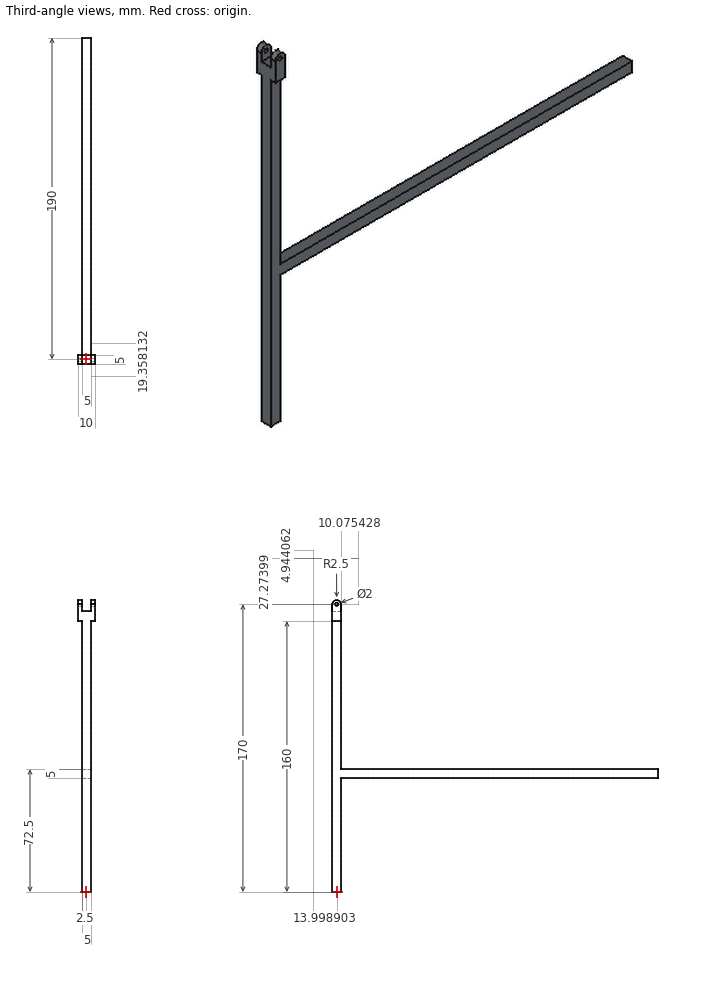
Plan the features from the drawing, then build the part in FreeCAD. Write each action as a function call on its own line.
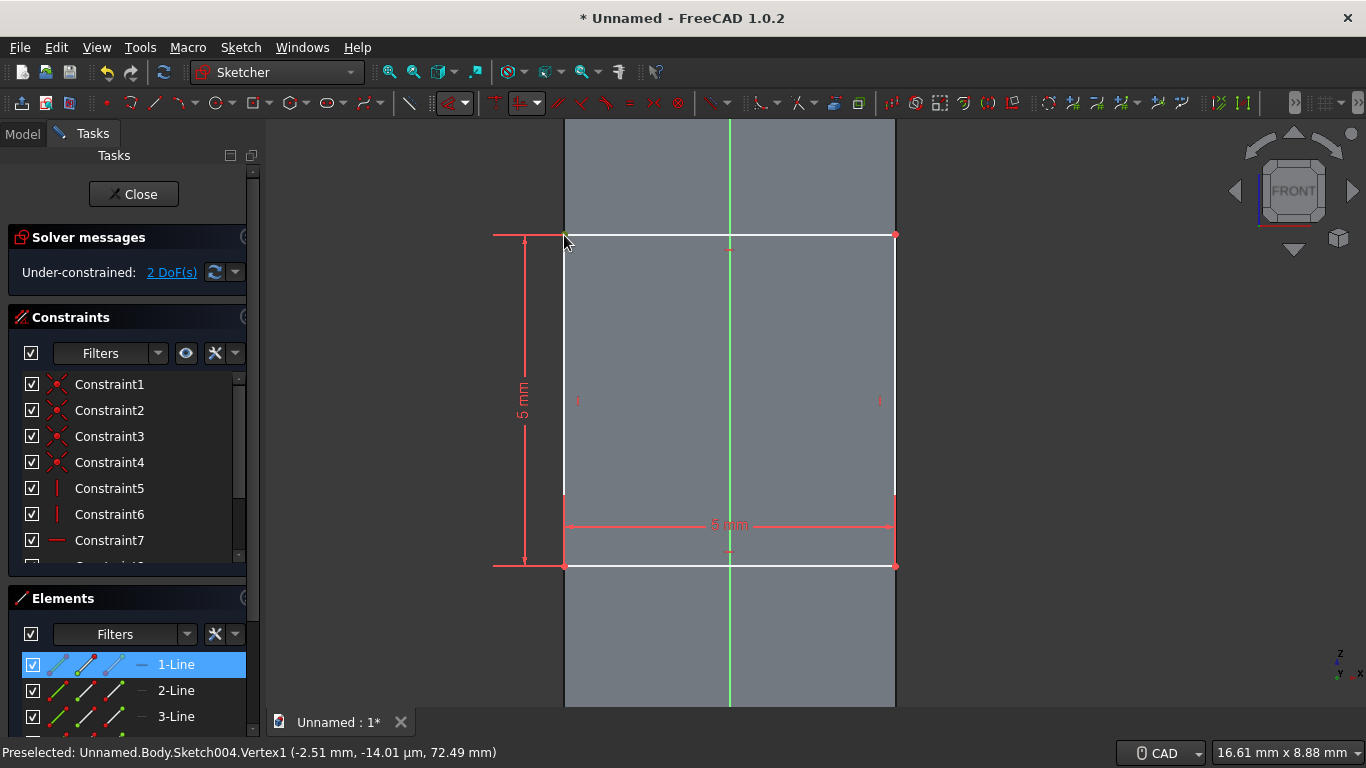
click(468, 104)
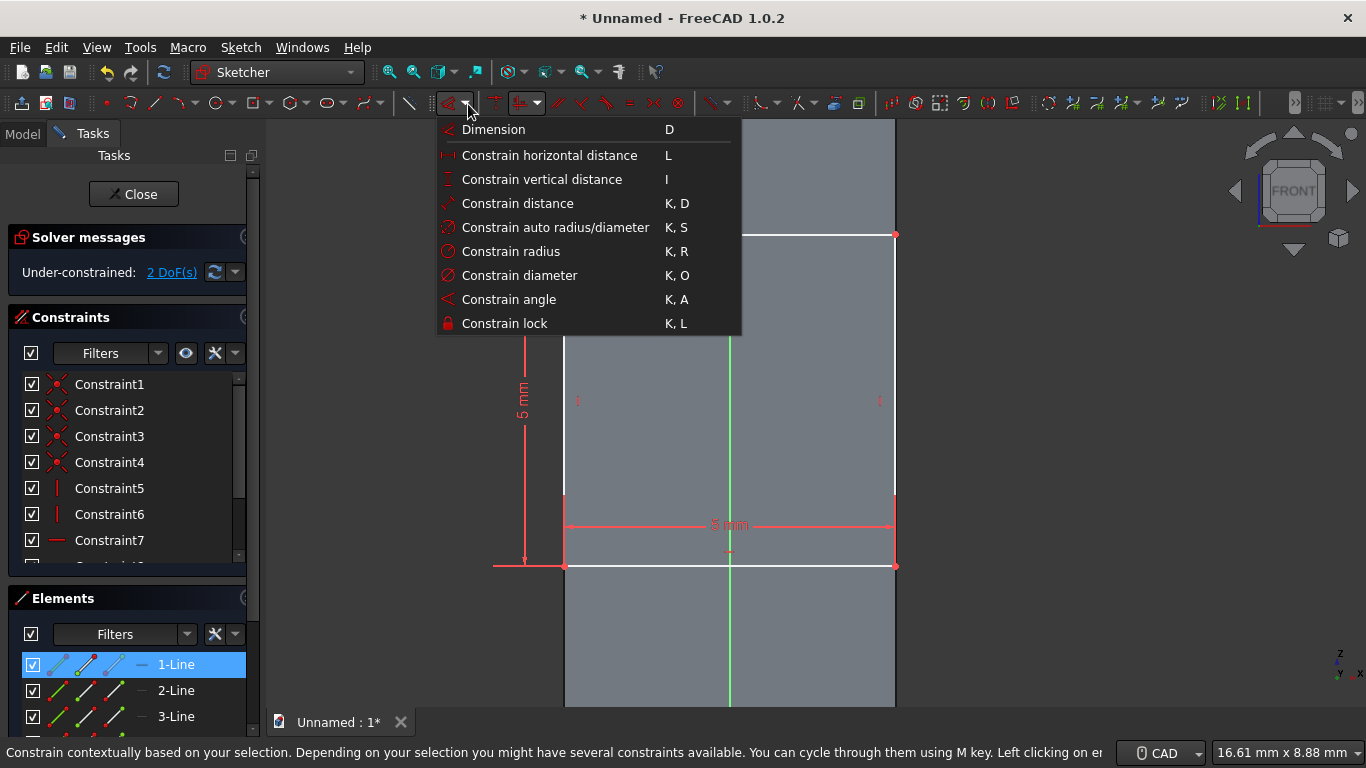
click(589, 155)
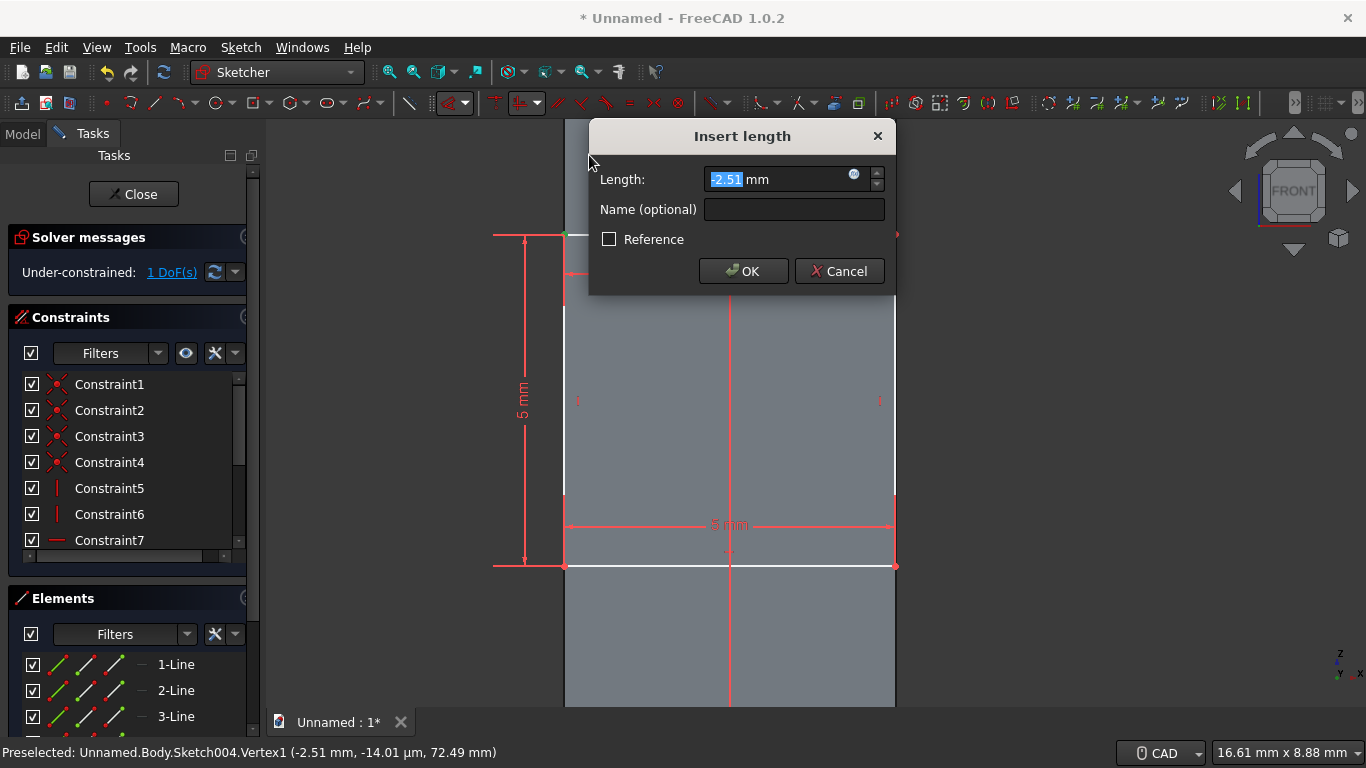
text(-2.5)
key(Return)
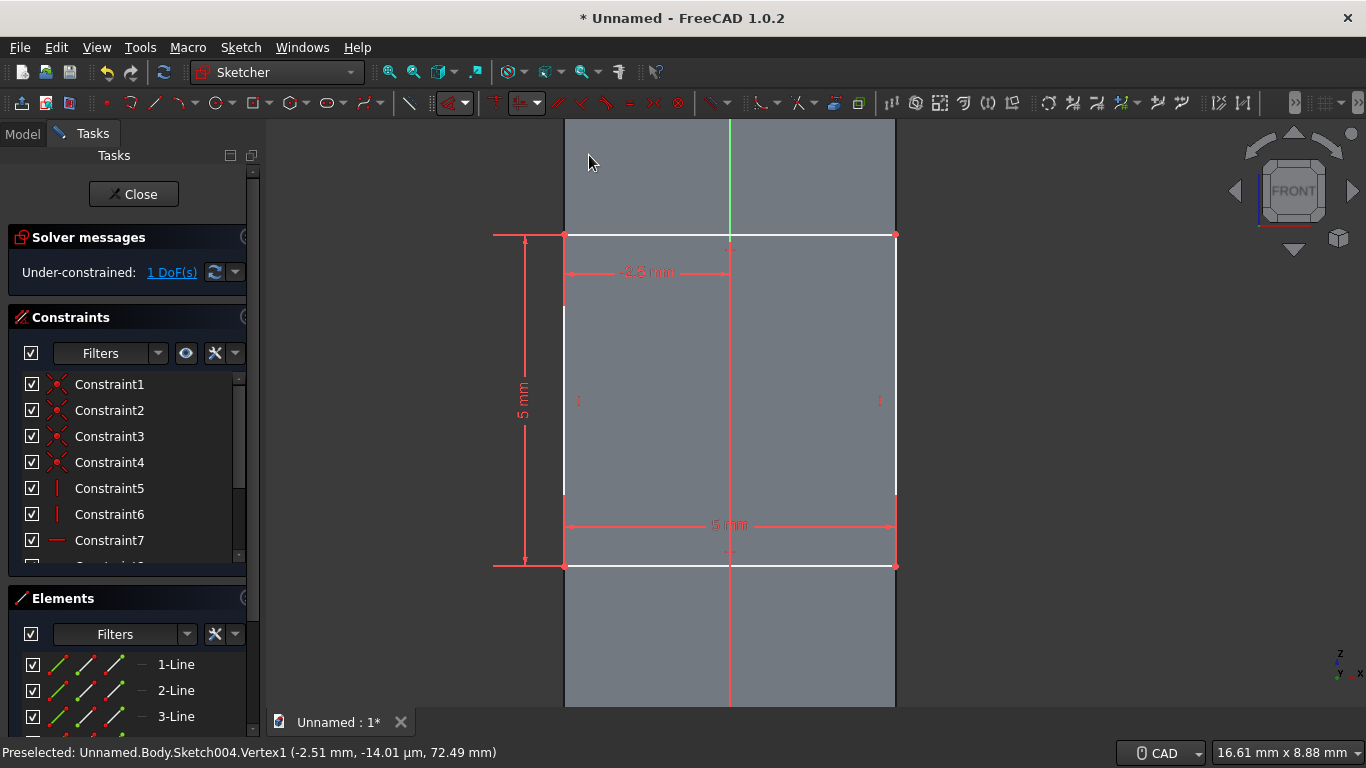
click(564, 235)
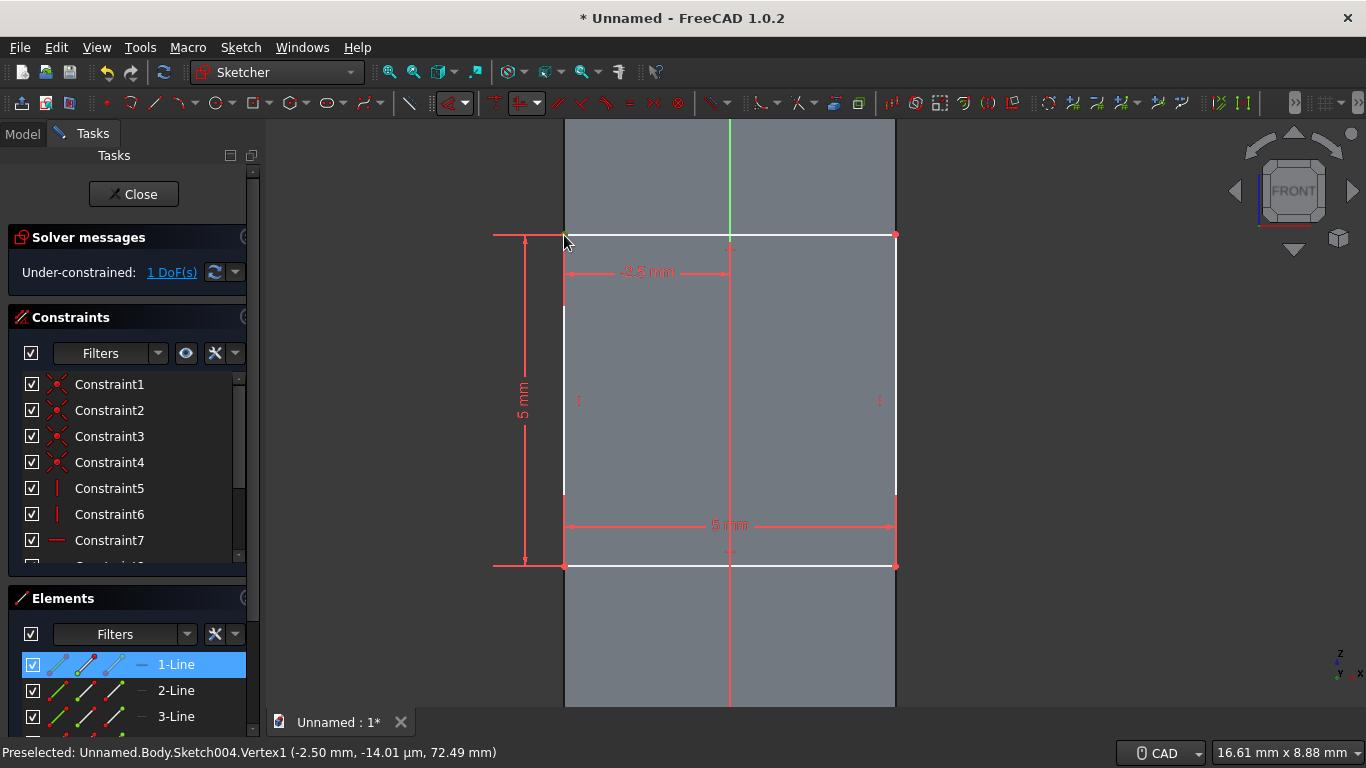
key(i)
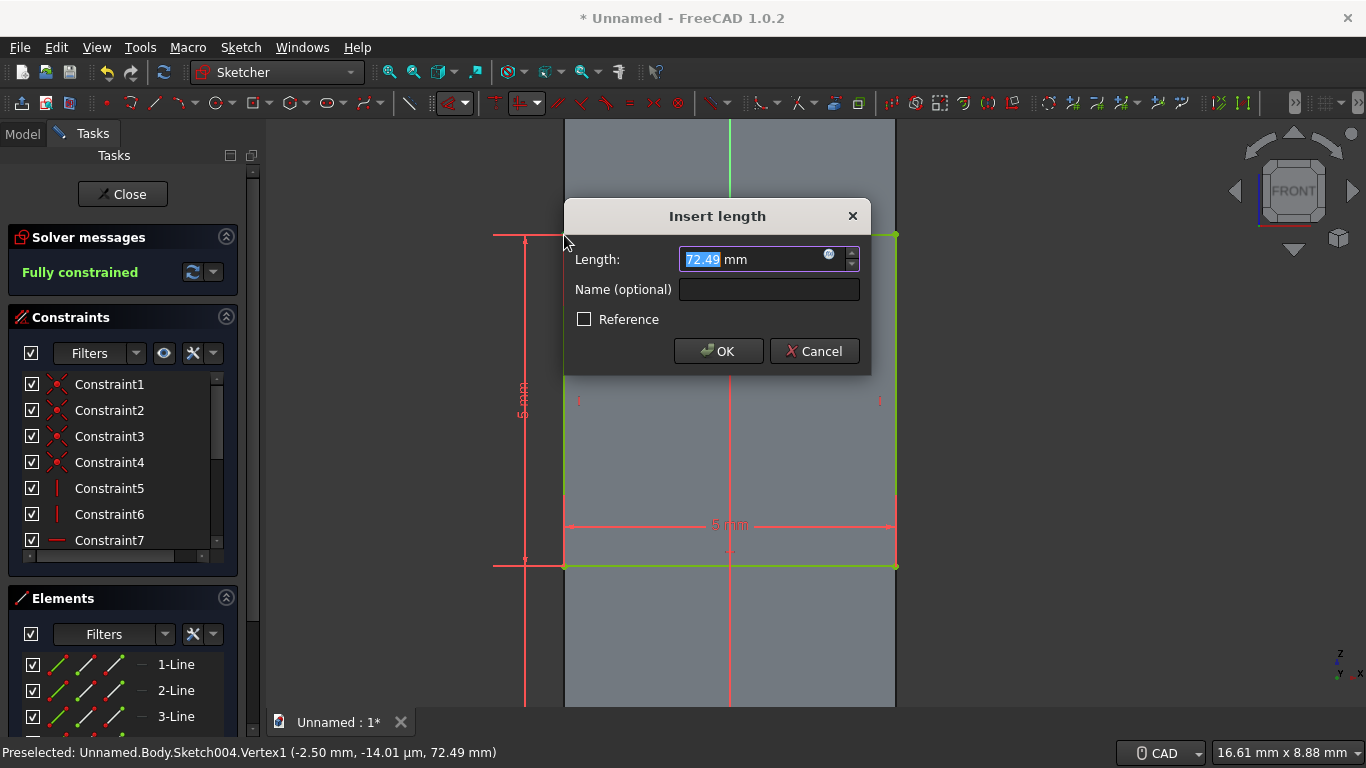
text(72.5)
key(Return)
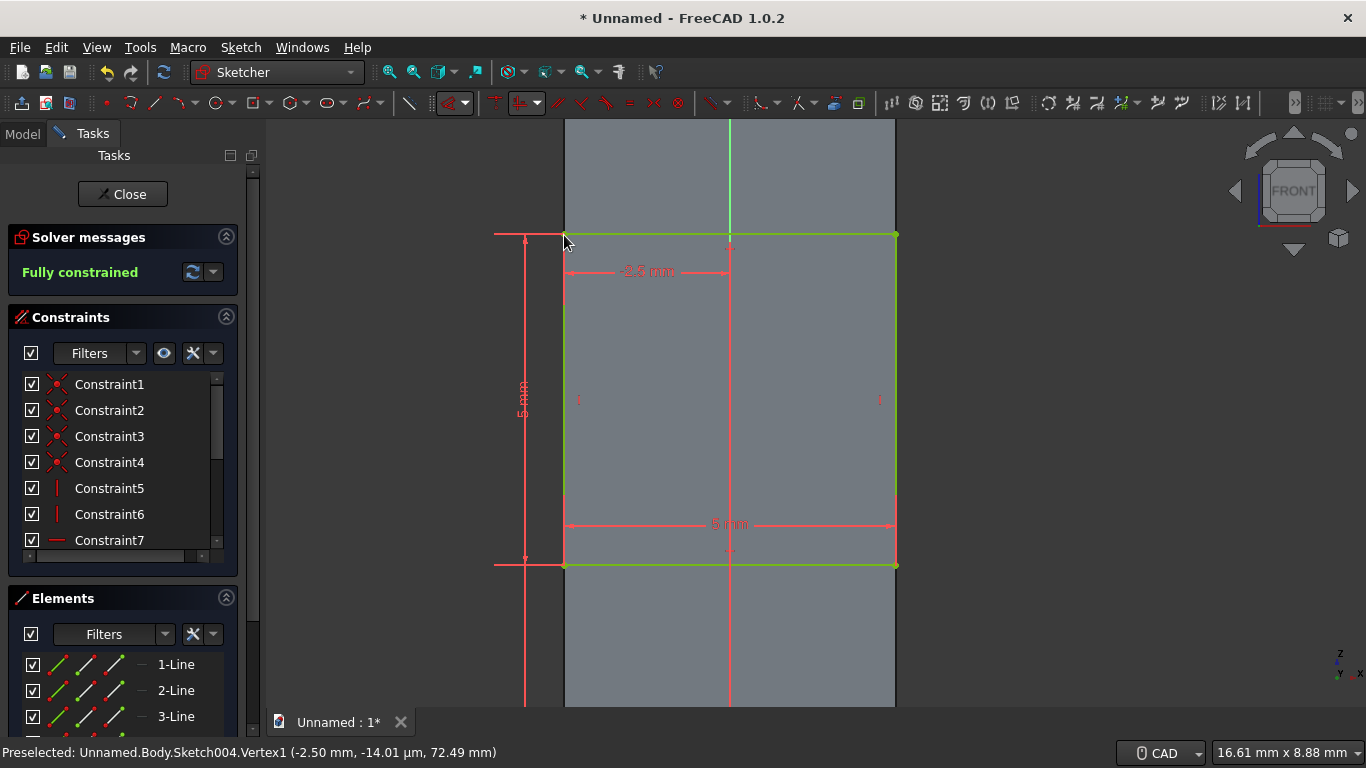
click(123, 194)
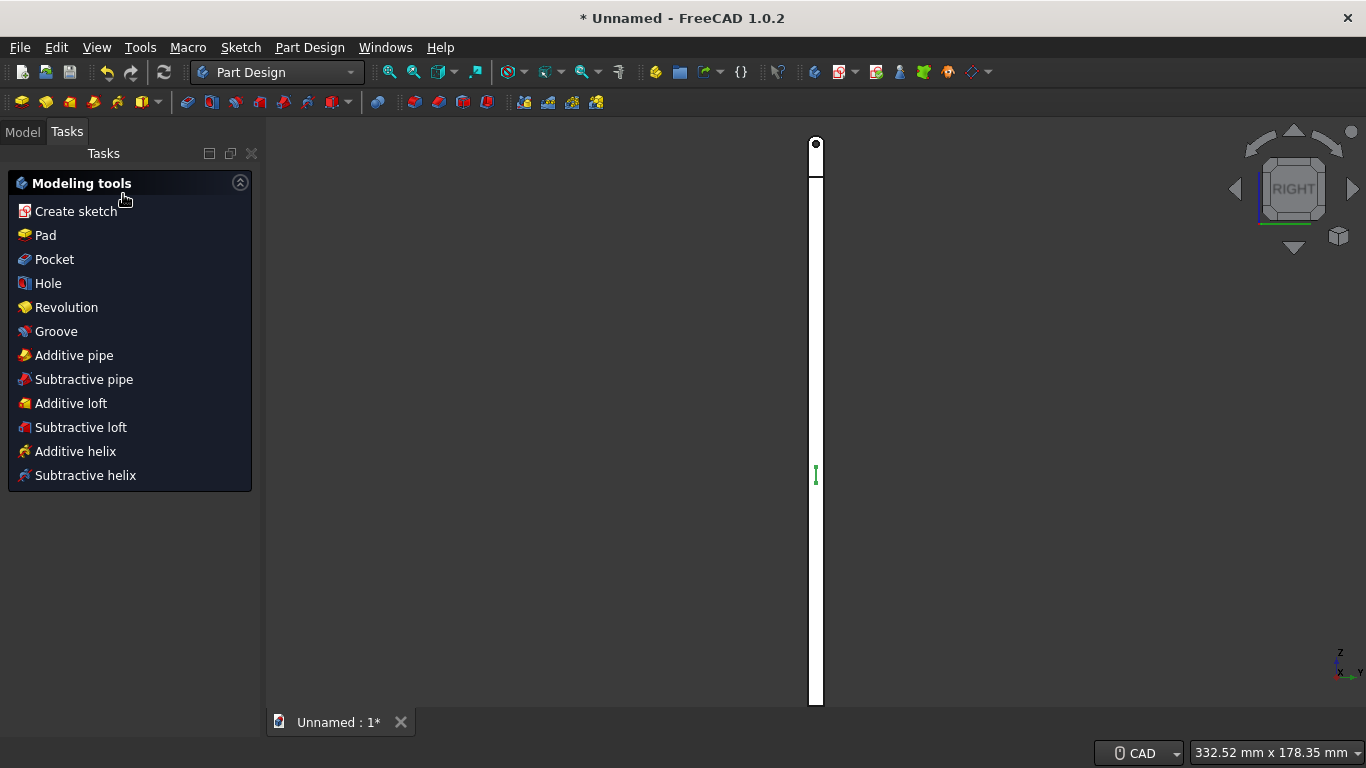
click(22, 102)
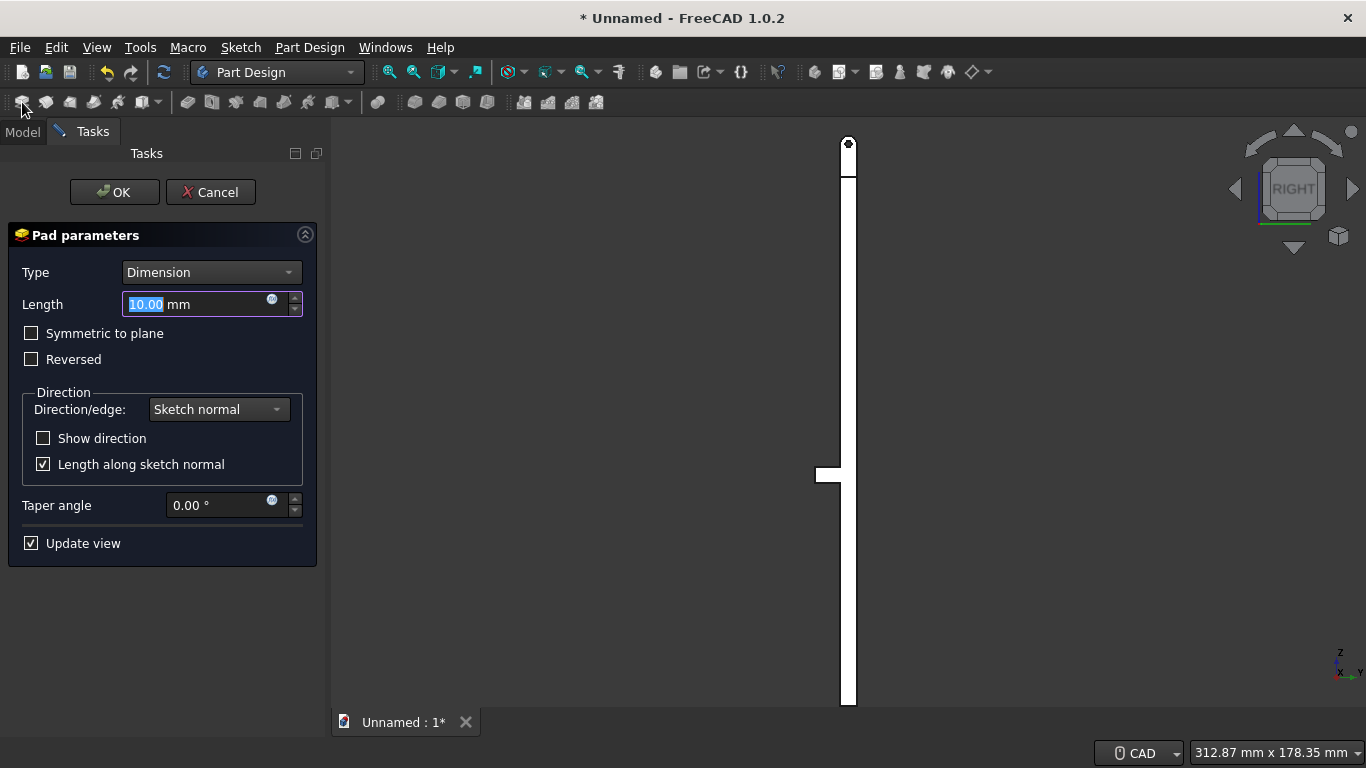
text(190)
key(Tab)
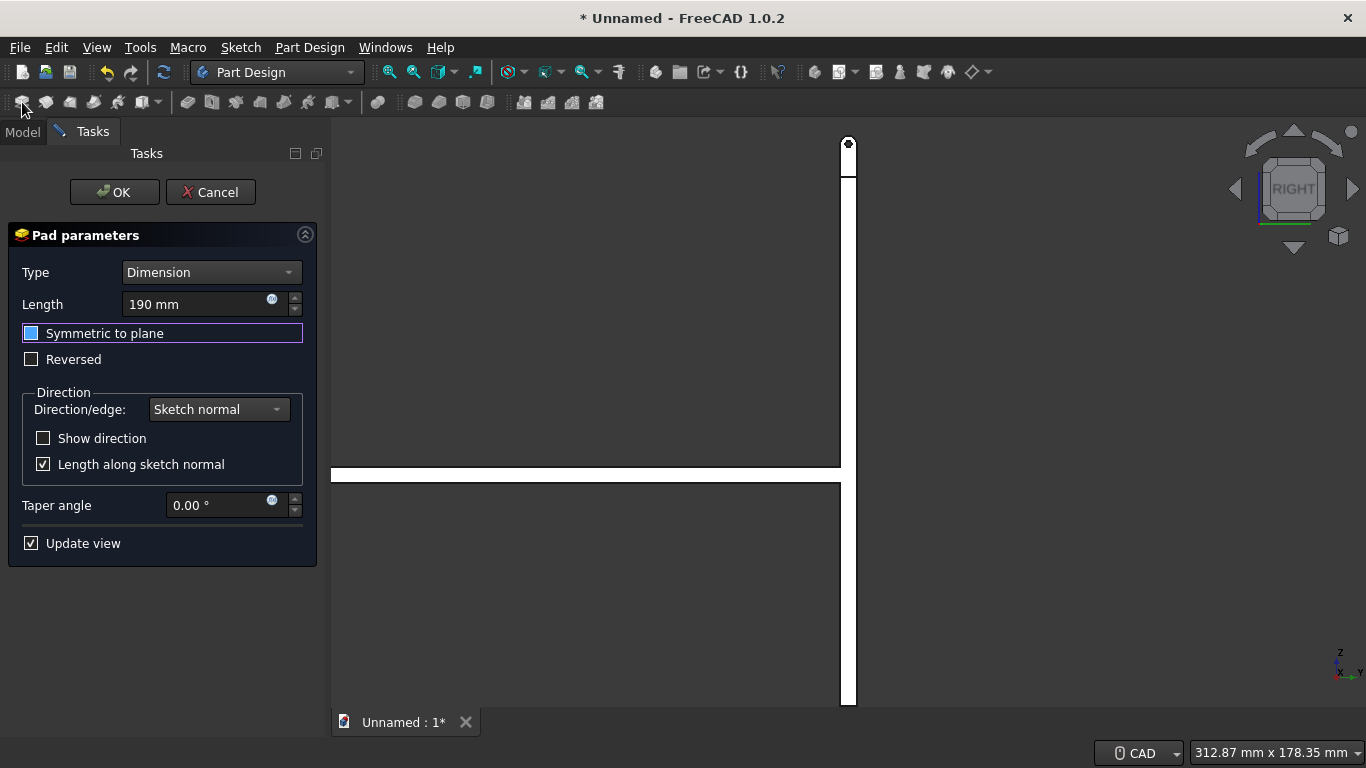
click(30, 359)